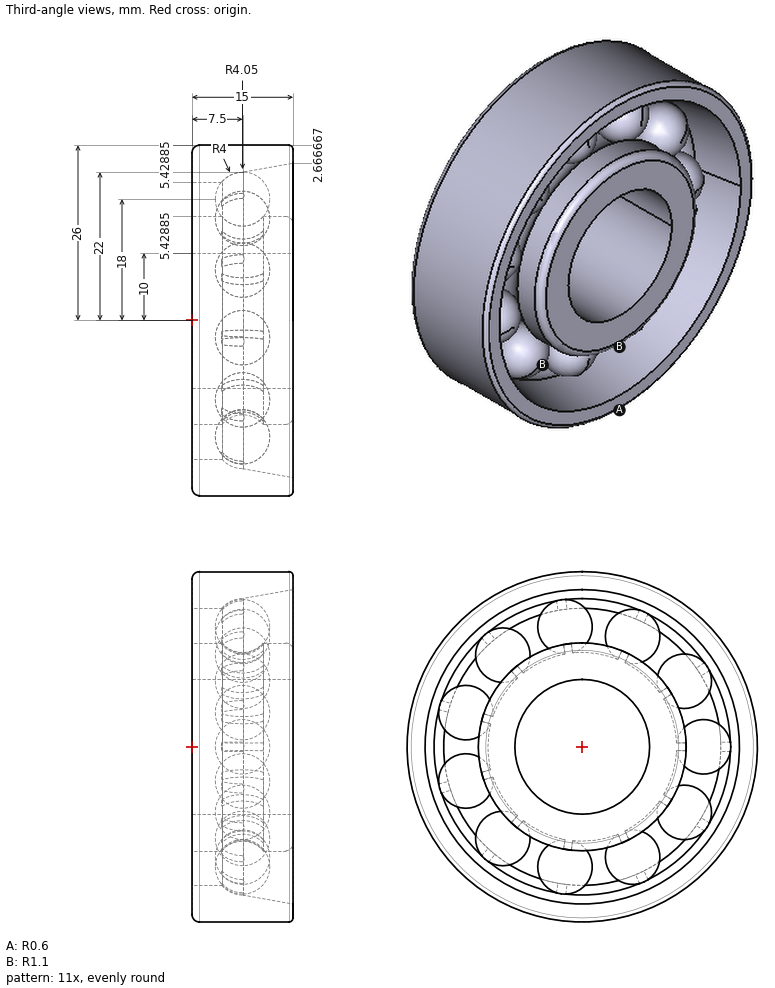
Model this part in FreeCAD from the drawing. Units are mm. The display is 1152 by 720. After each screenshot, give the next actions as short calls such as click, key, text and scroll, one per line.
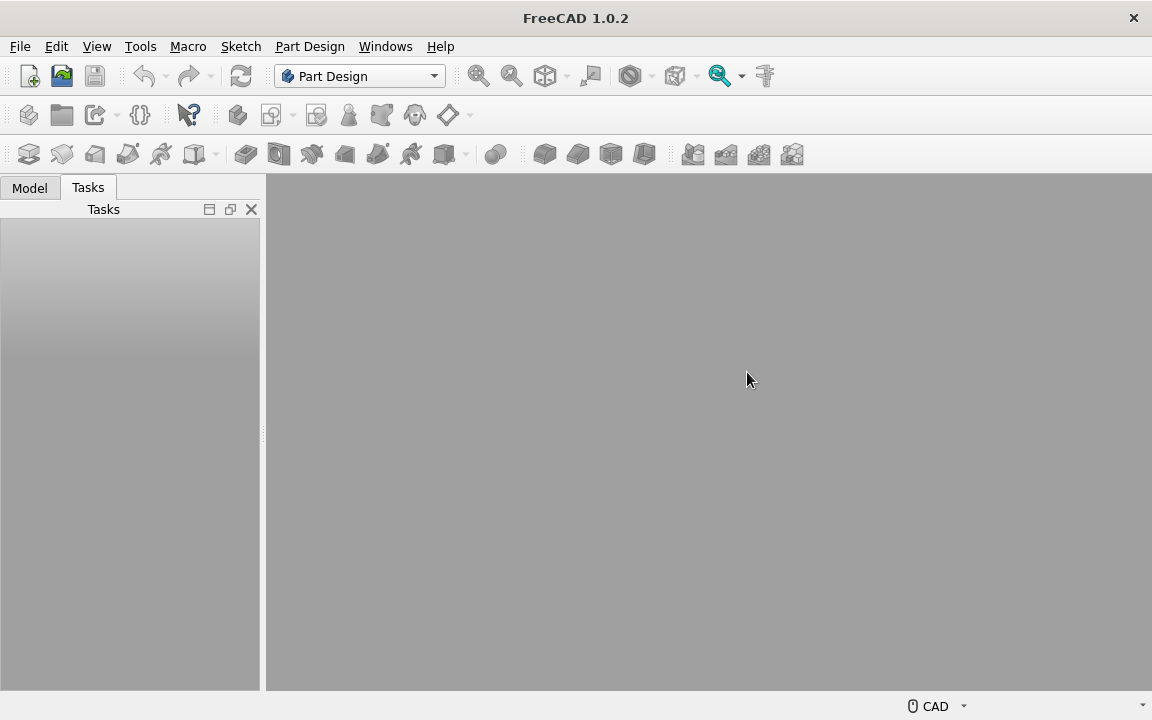
click(29, 76)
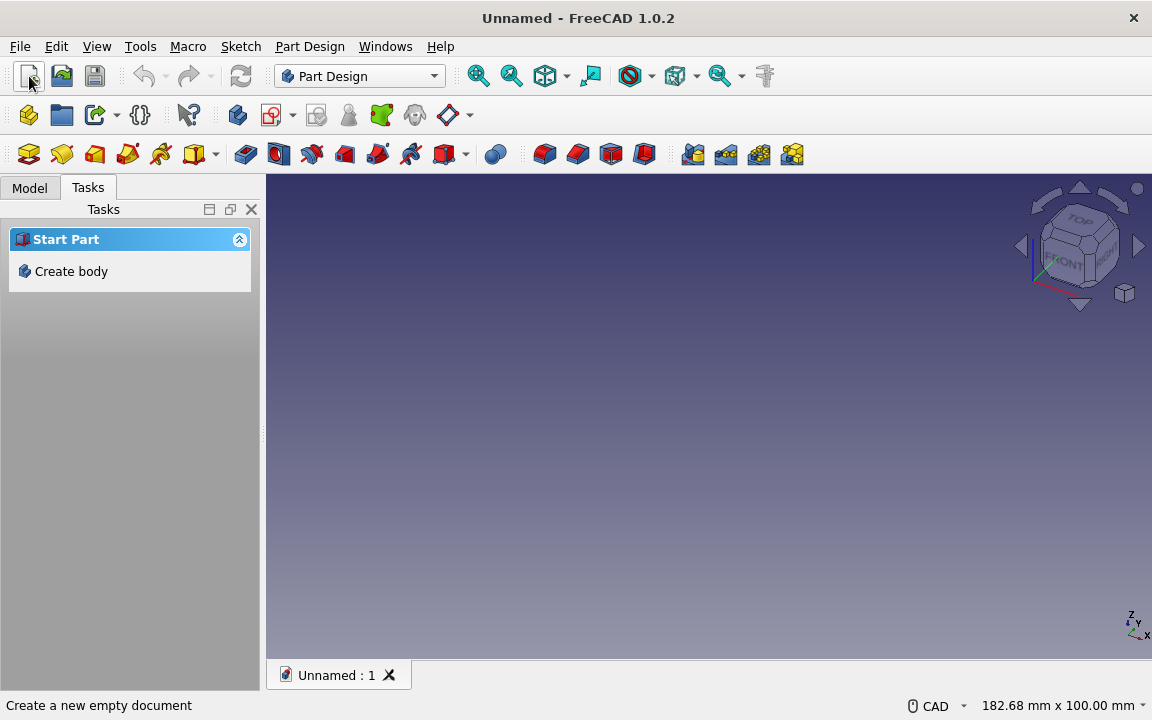
click(270, 116)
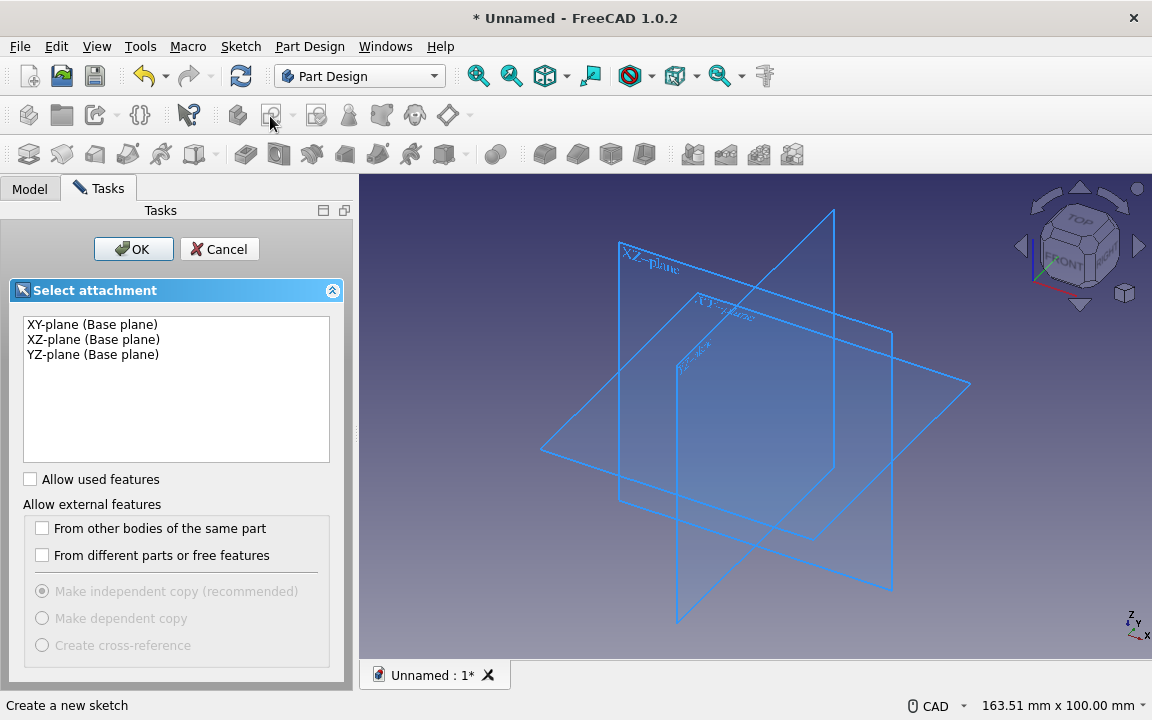
click(84, 324)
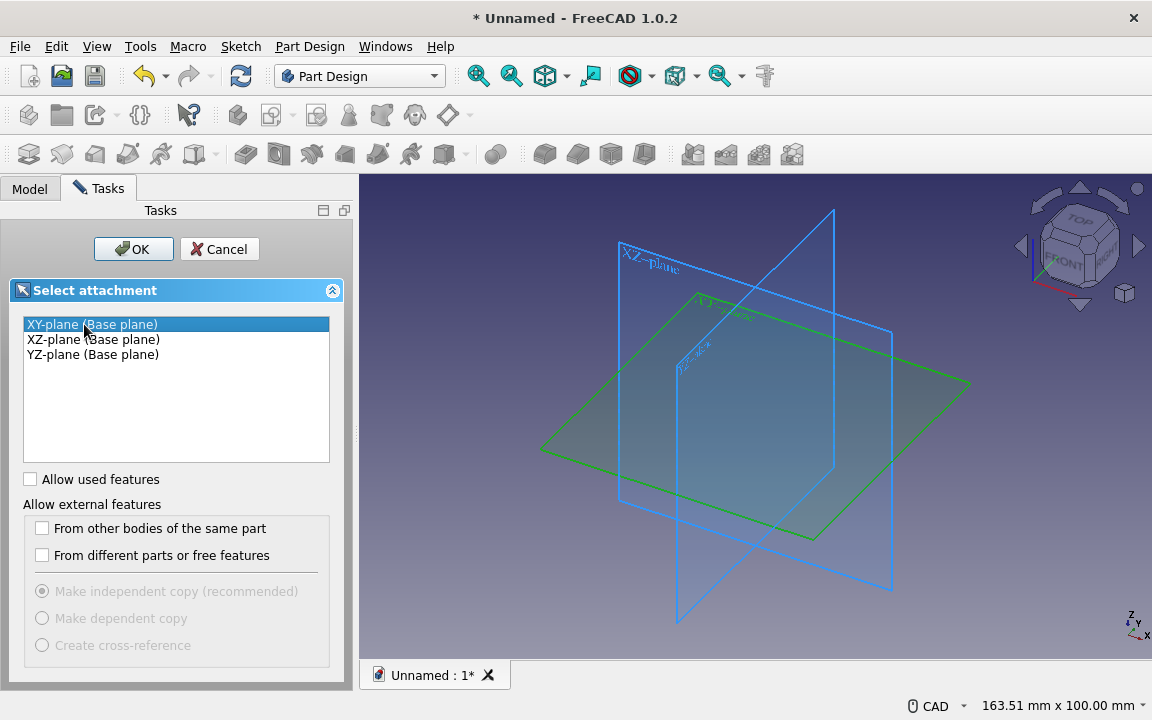
click(134, 249)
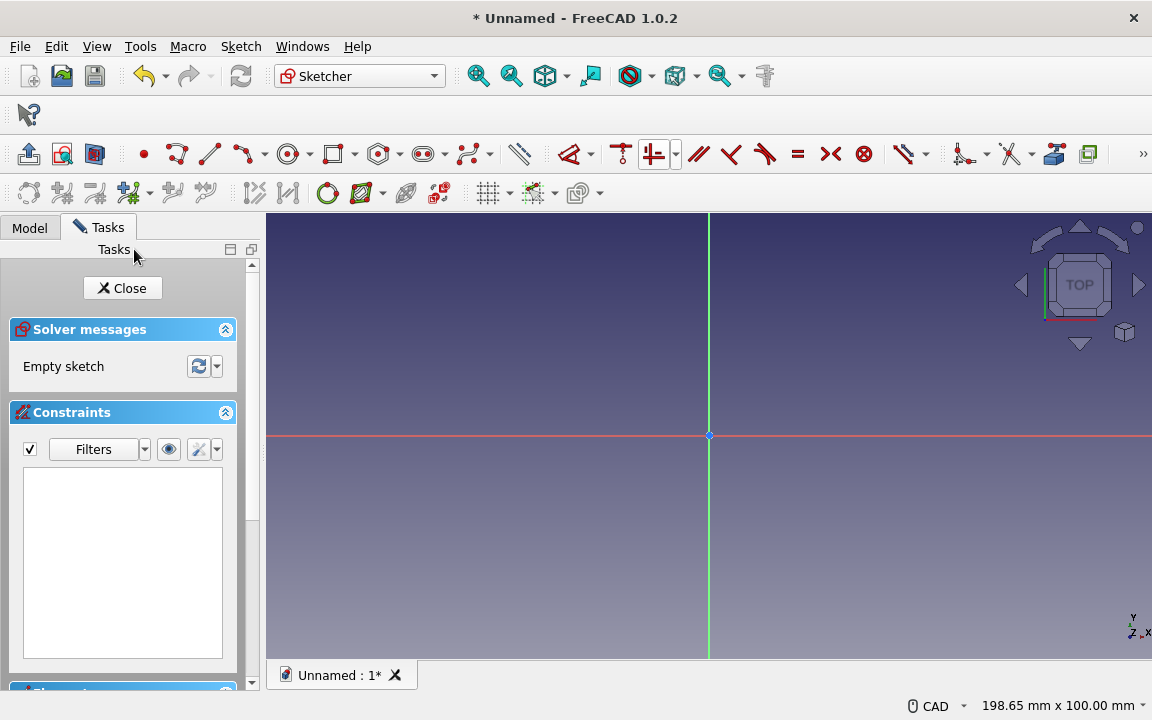
scroll(826, 331, up, 4)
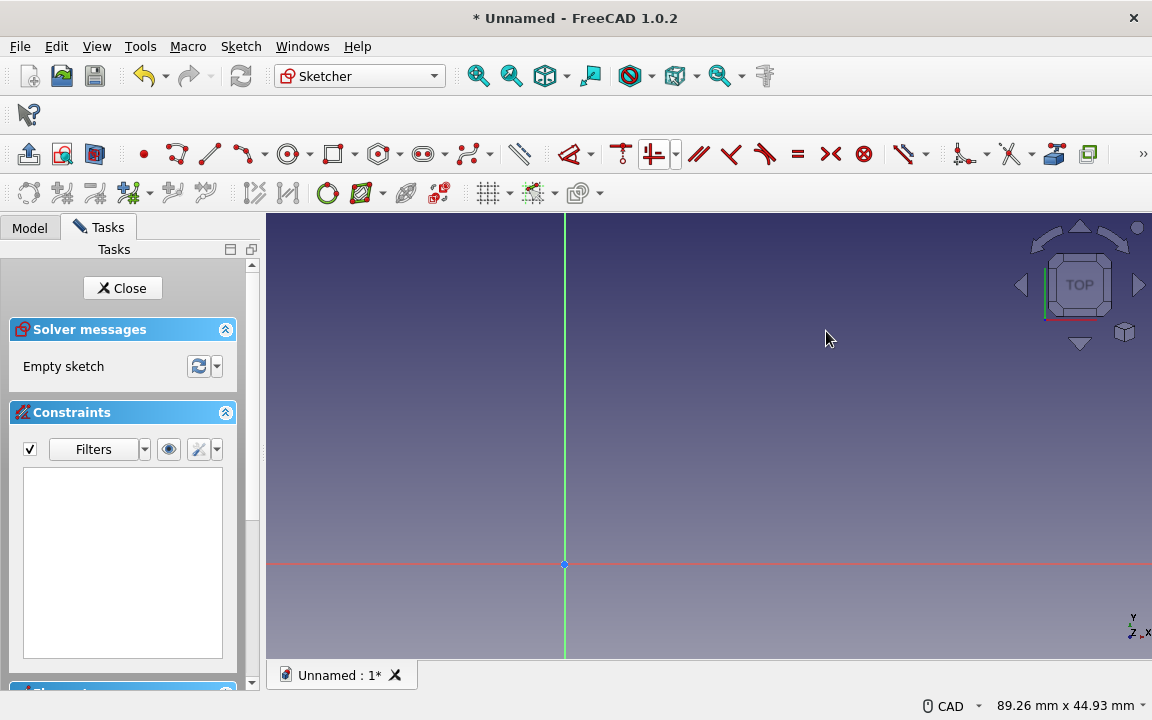
key(g)
key(m)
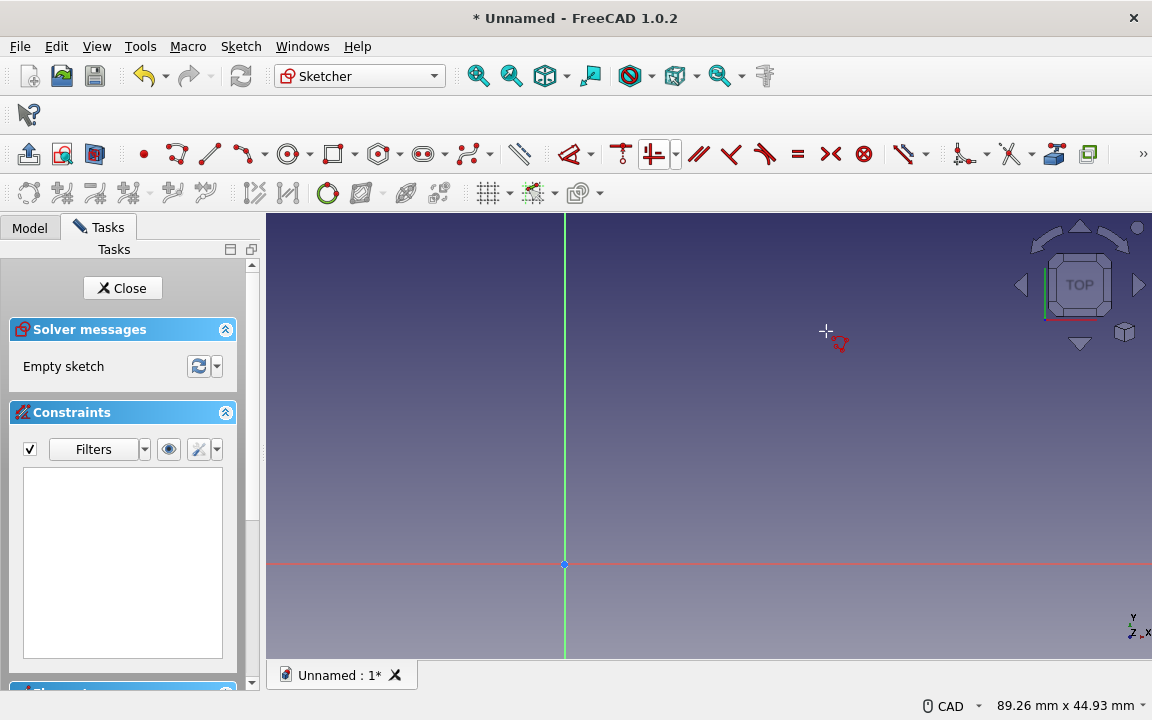
click(639, 346)
click(714, 333)
click(714, 306)
click(565, 306)
click(574, 360)
click(609, 360)
right_click(609, 360)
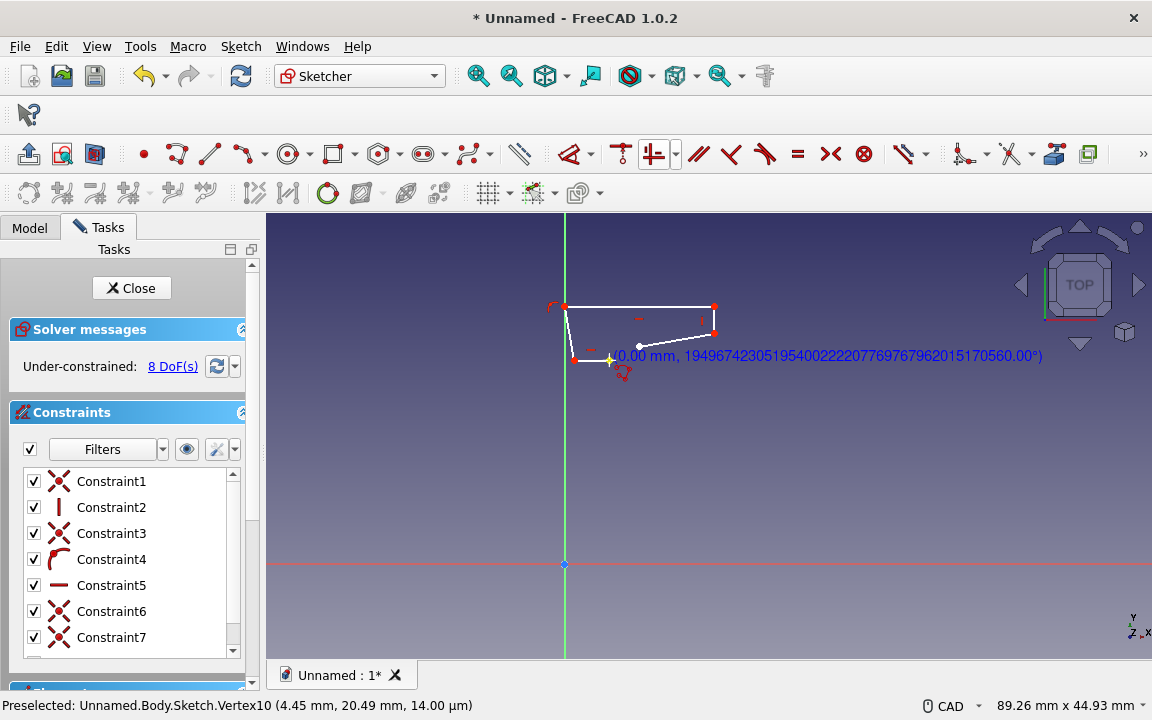
click(242, 154)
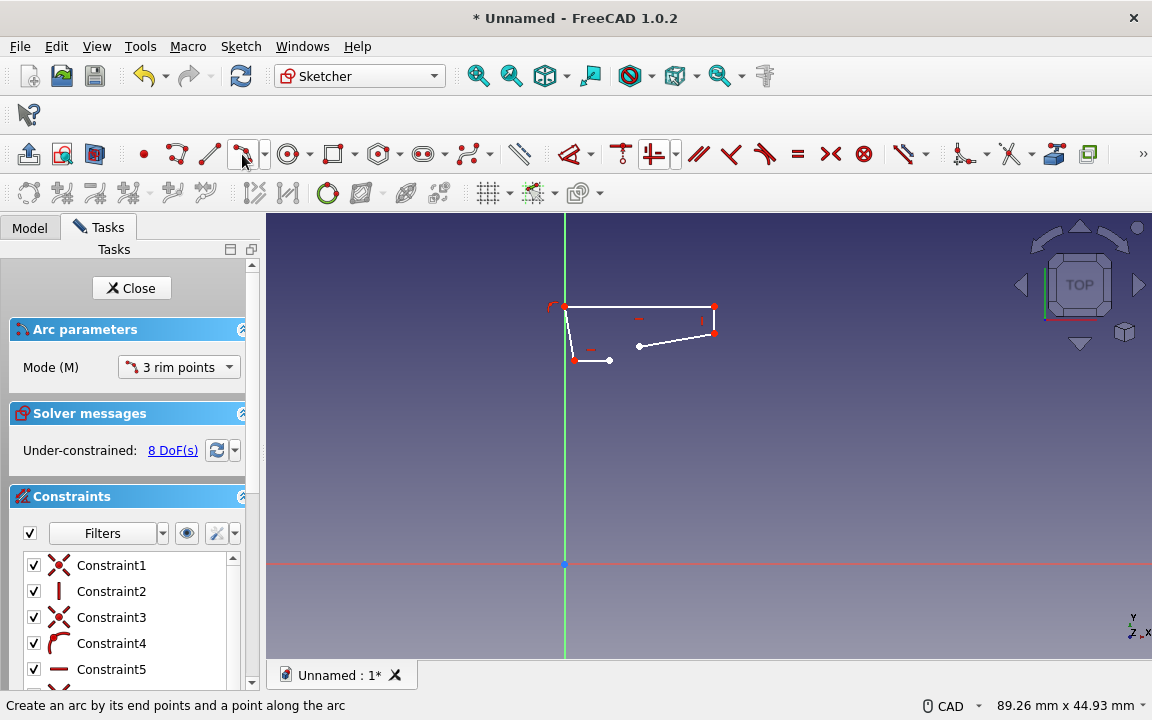
click(609, 361)
click(639, 347)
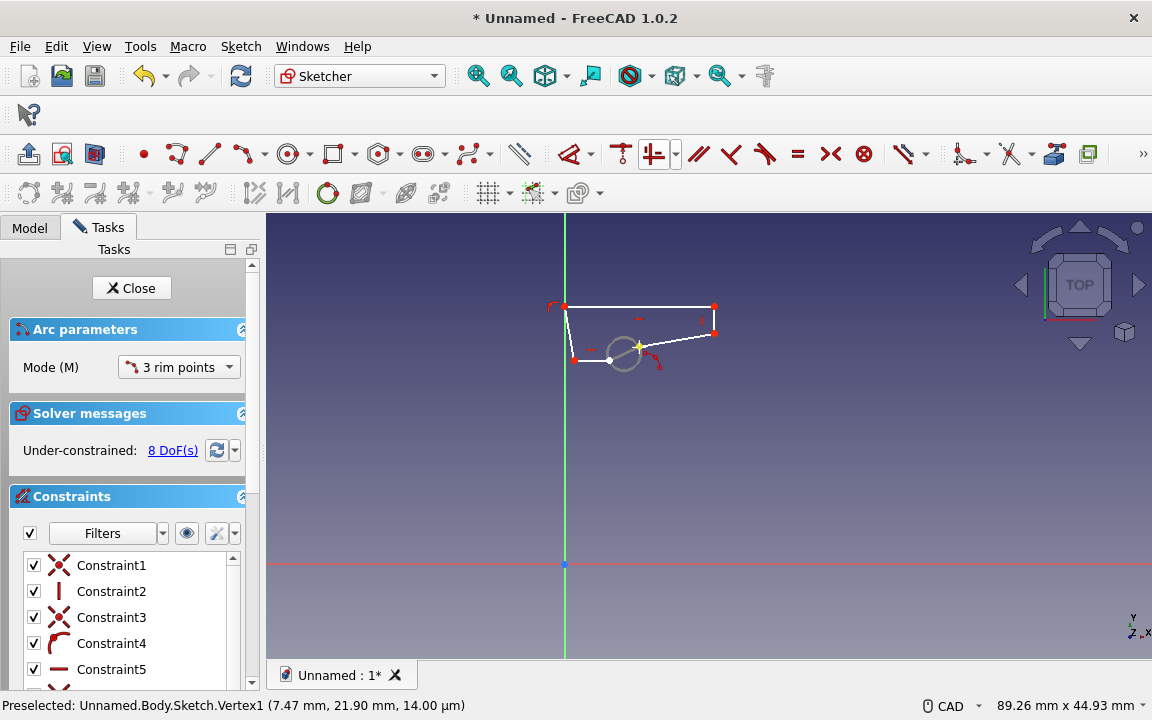
scroll(623, 350, up, 8)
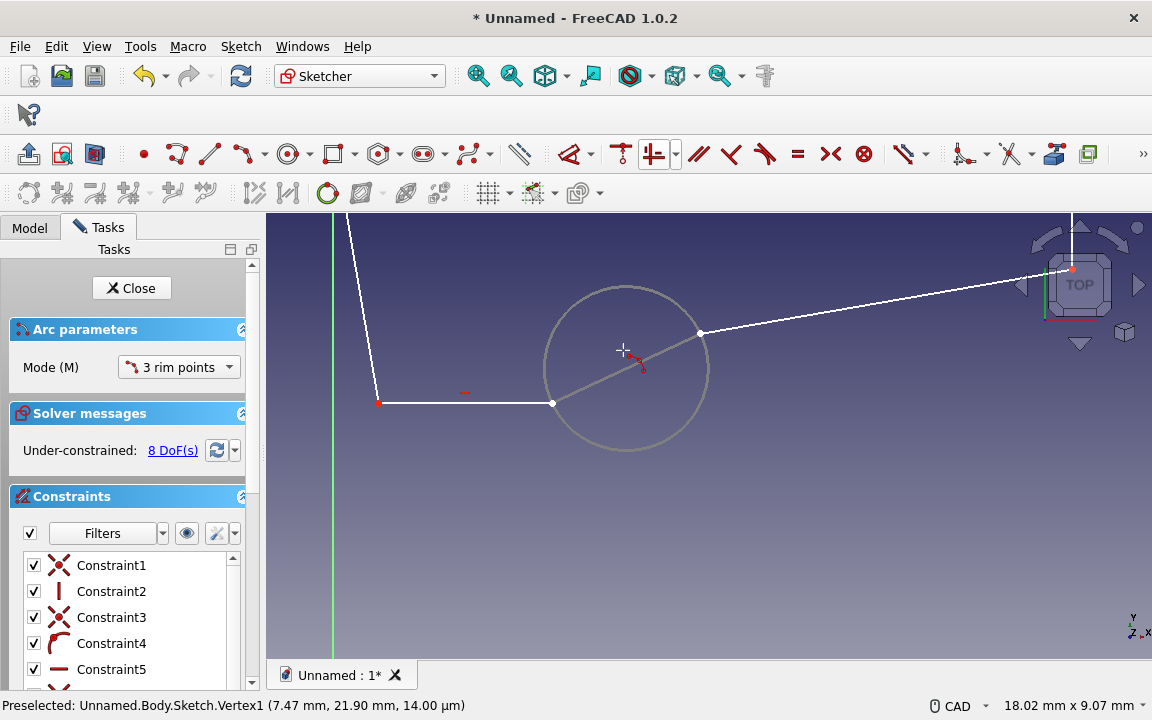
click(619, 347)
key(Escape)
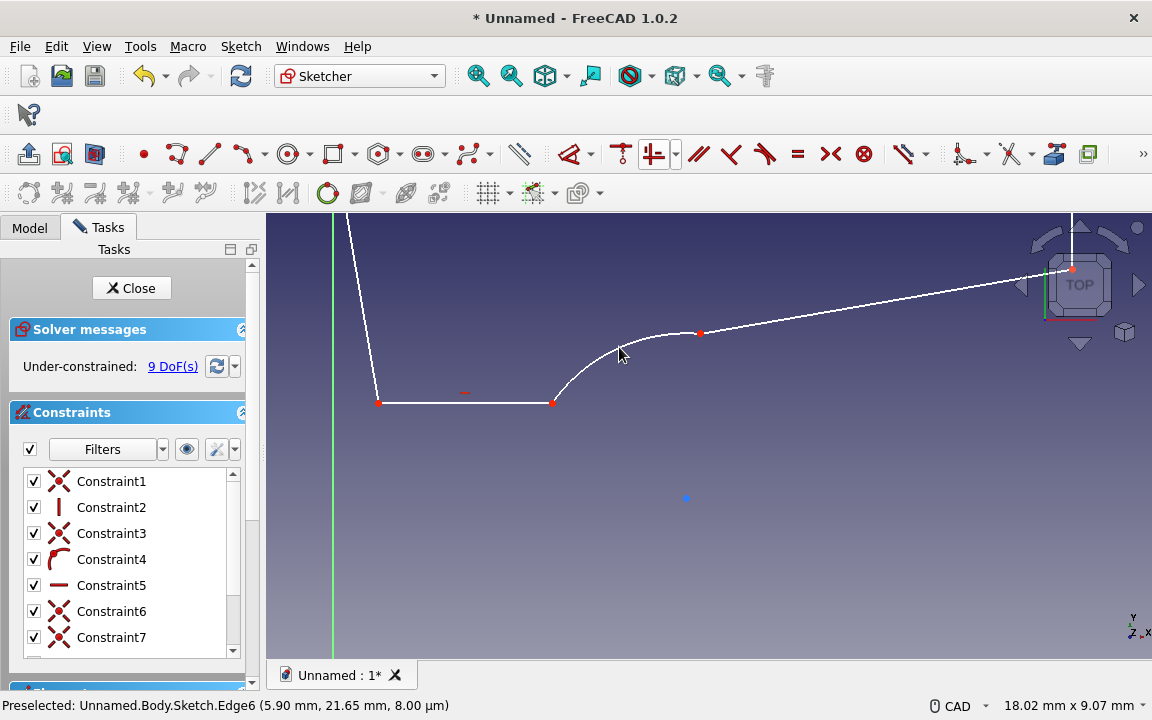
click(365, 323)